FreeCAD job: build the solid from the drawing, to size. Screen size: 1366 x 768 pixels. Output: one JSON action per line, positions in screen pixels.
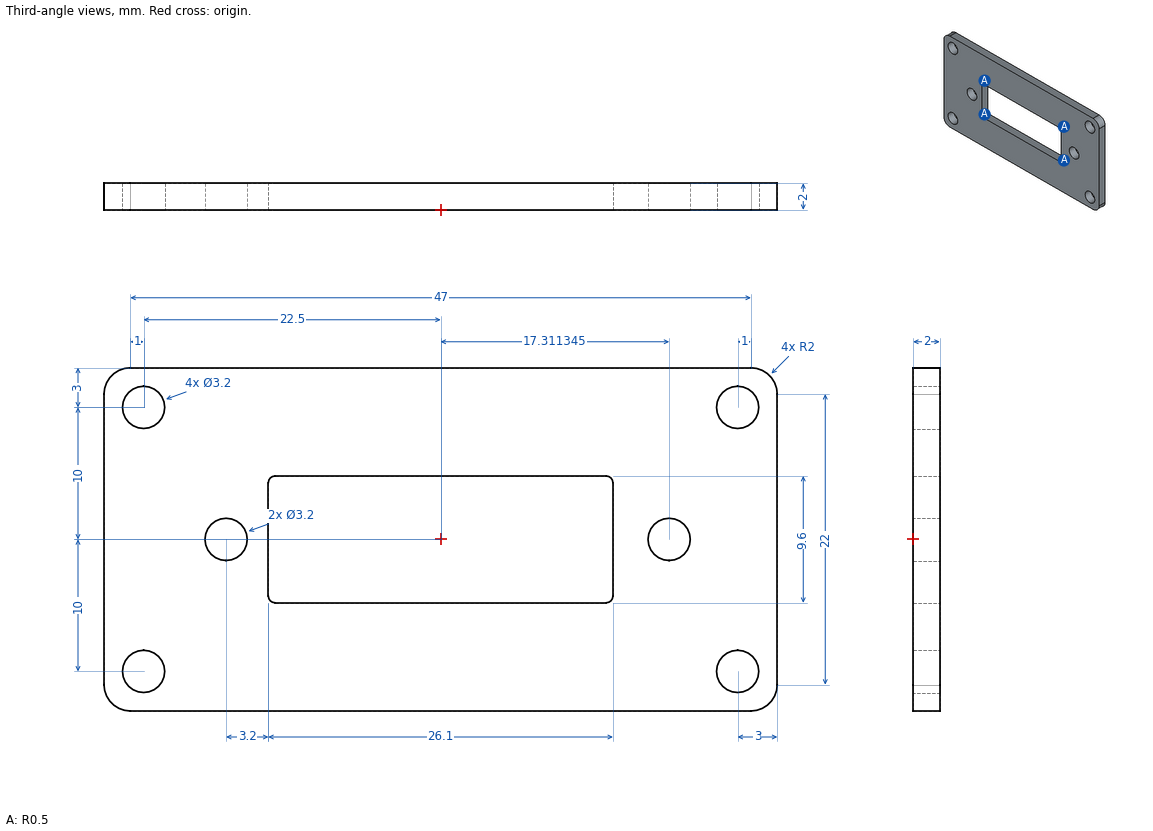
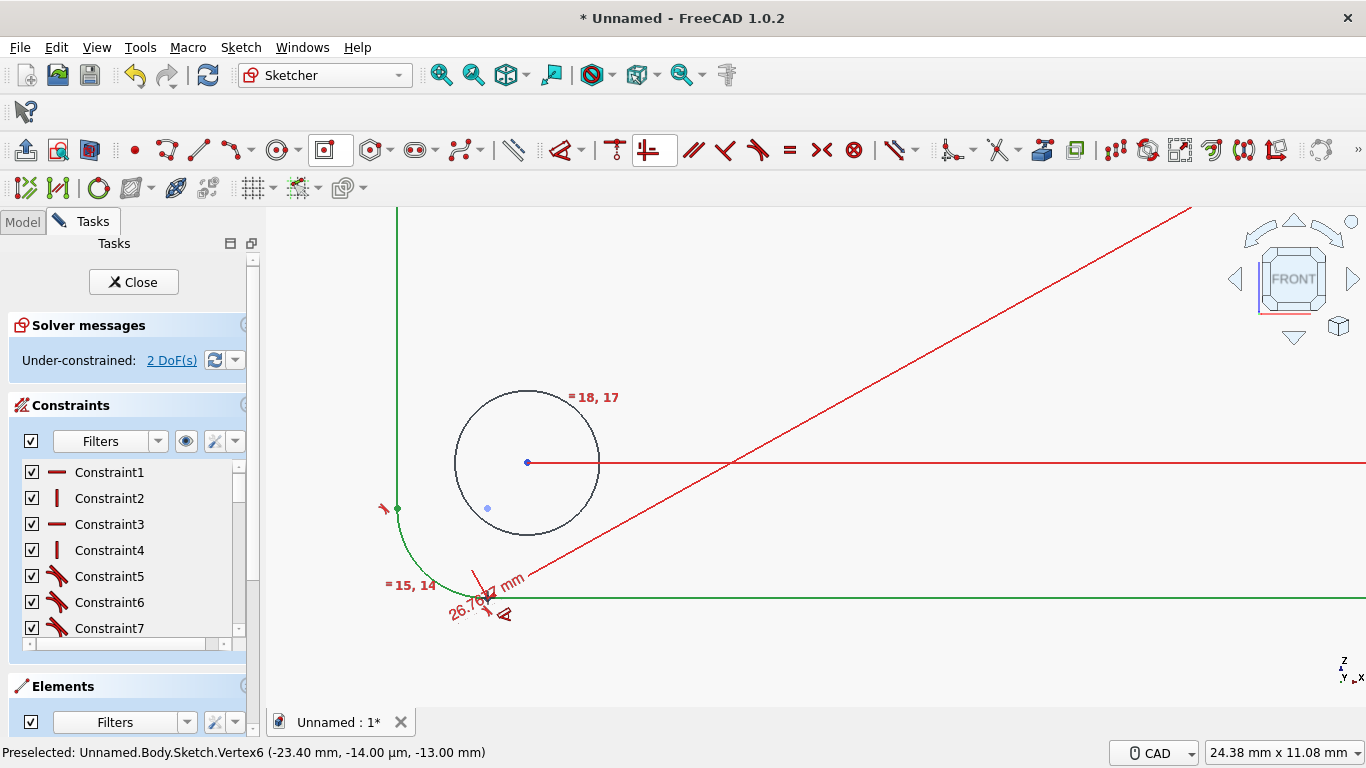
{"action": "left_click", "coordinate": [527, 463]}
{"action": "left_click", "coordinate": [507, 632]}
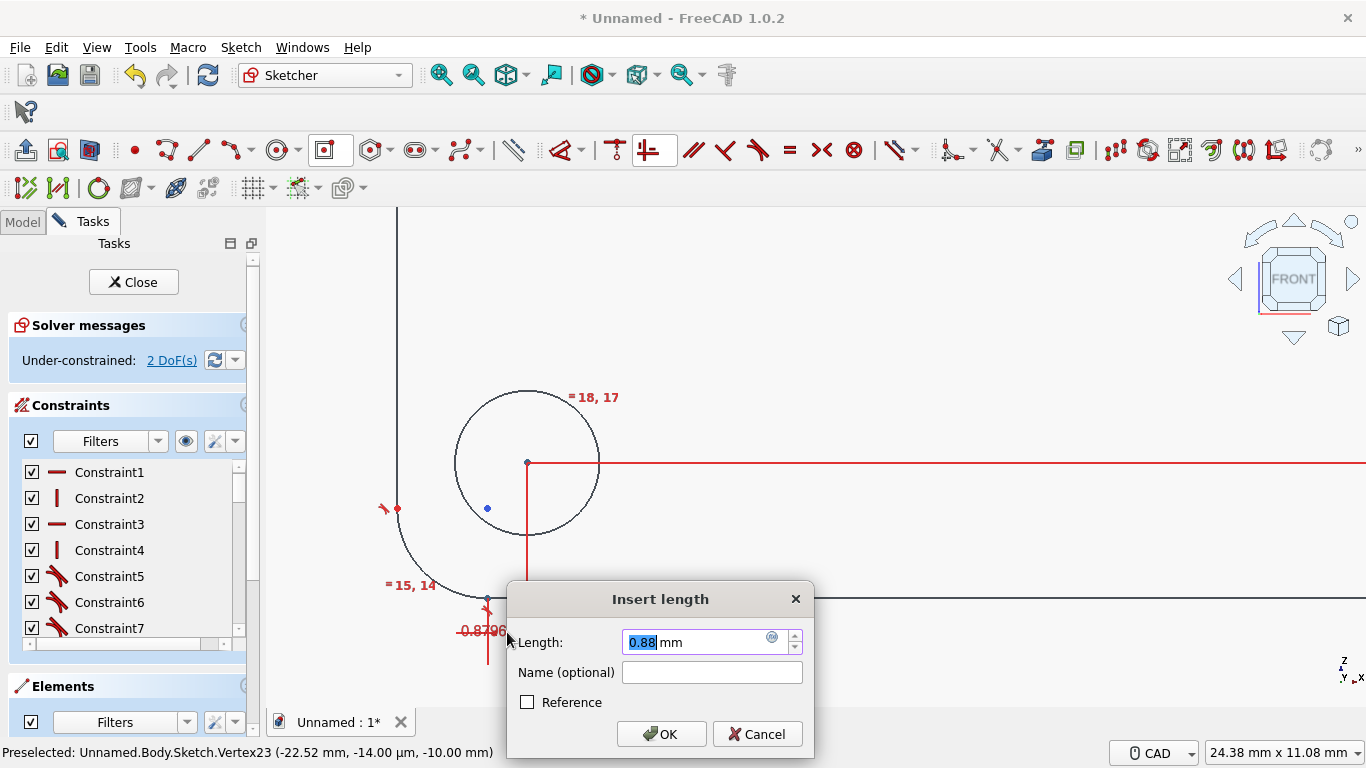
{"action": "type", "text": "1"}
{"action": "key", "text": "Return"}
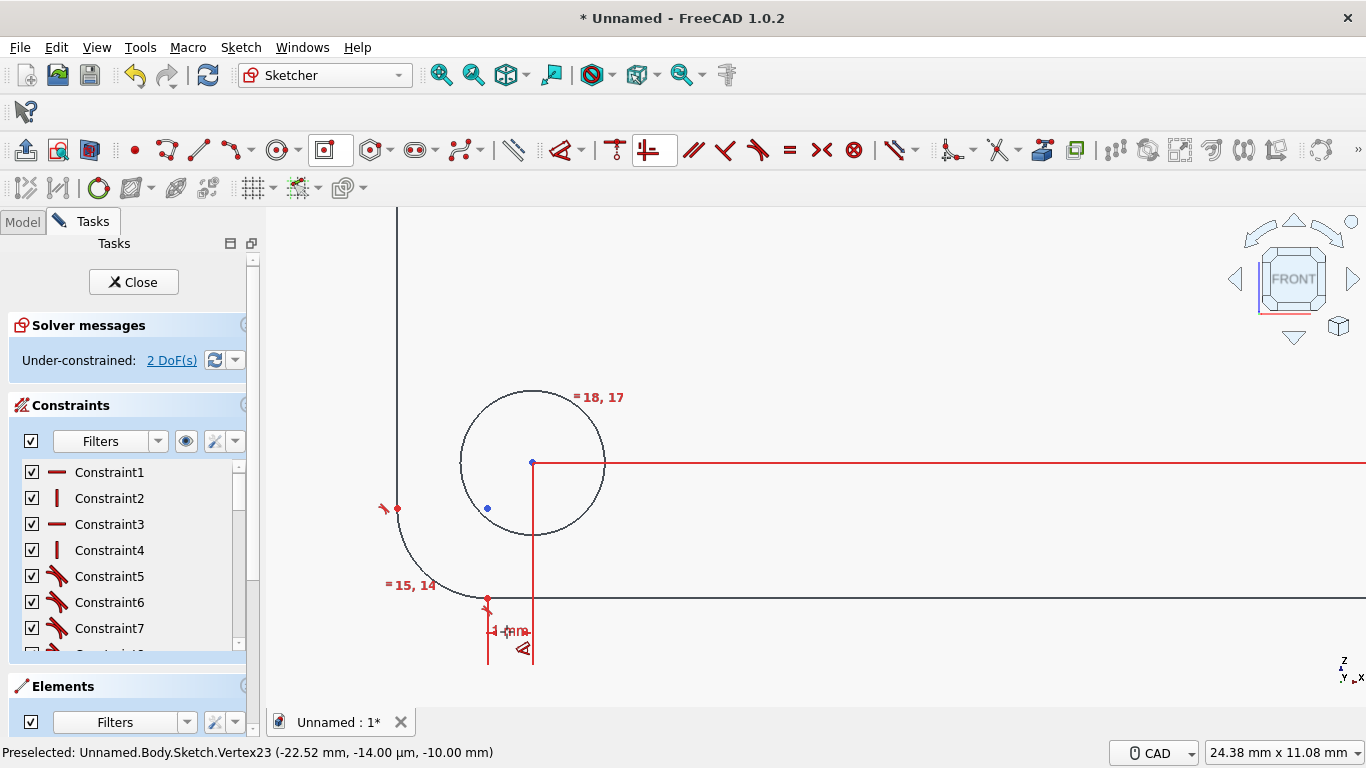
{"action": "scroll", "coordinate": [487, 603], "scroll_direction": "down", "scroll_amount": 7}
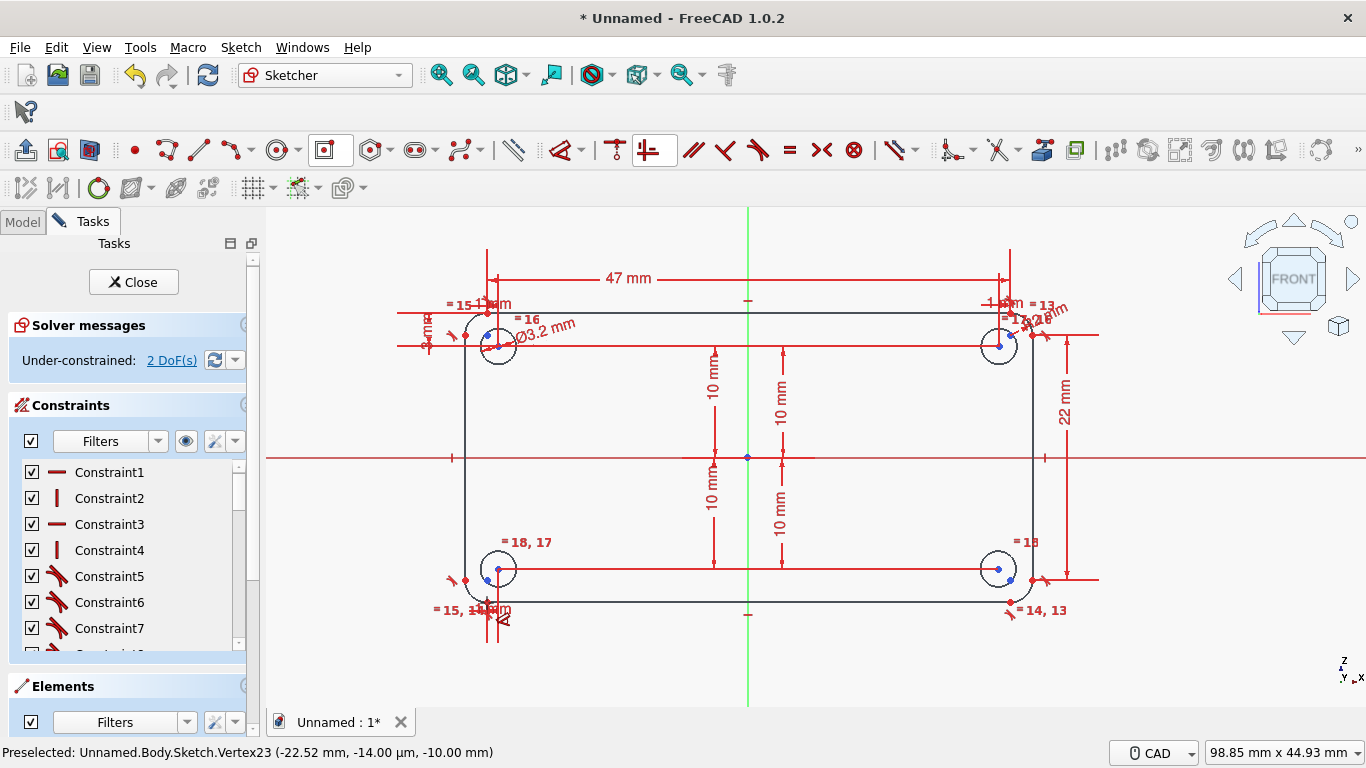
{"action": "left_click", "coordinate": [1033, 580]}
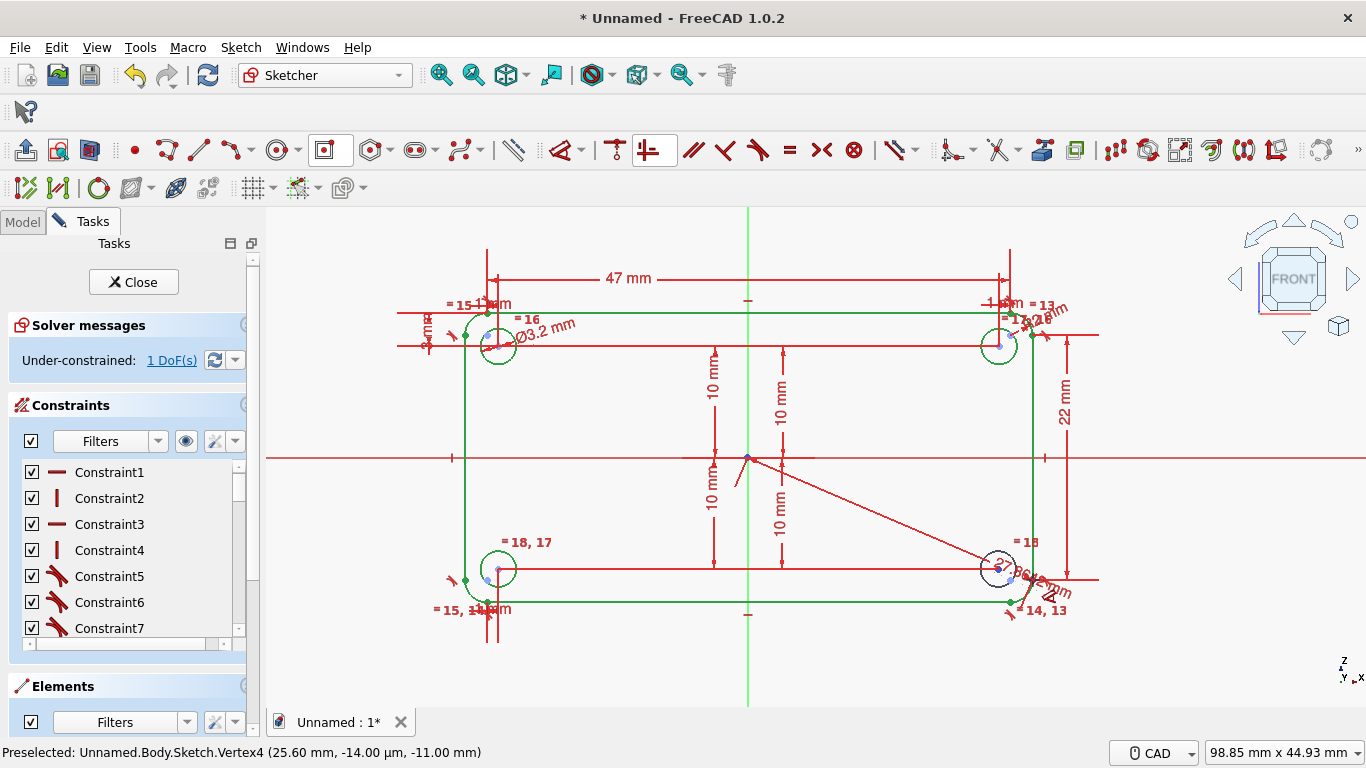
{"action": "left_click", "coordinate": [998, 569]}
{"action": "left_click", "coordinate": [1023, 614]}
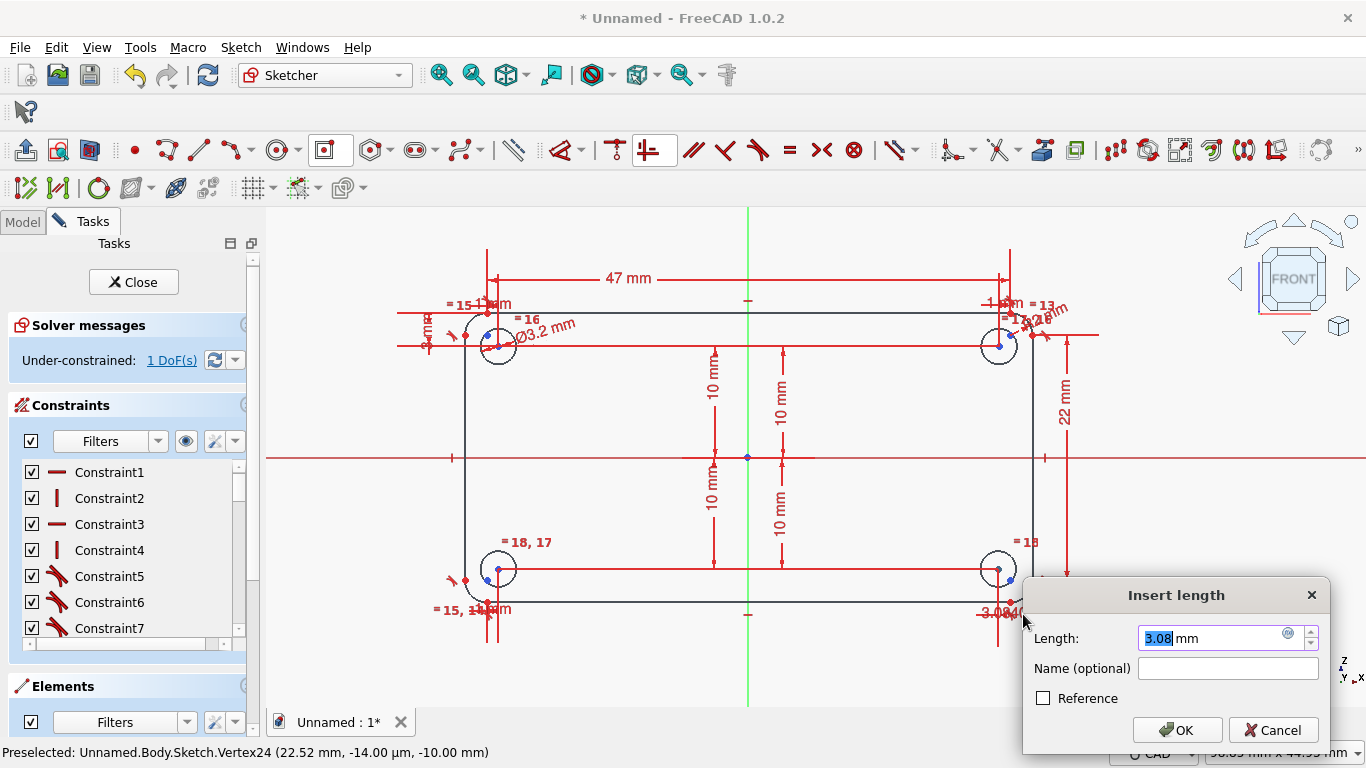
{"action": "type", "text": "3"}
{"action": "key", "text": "Return"}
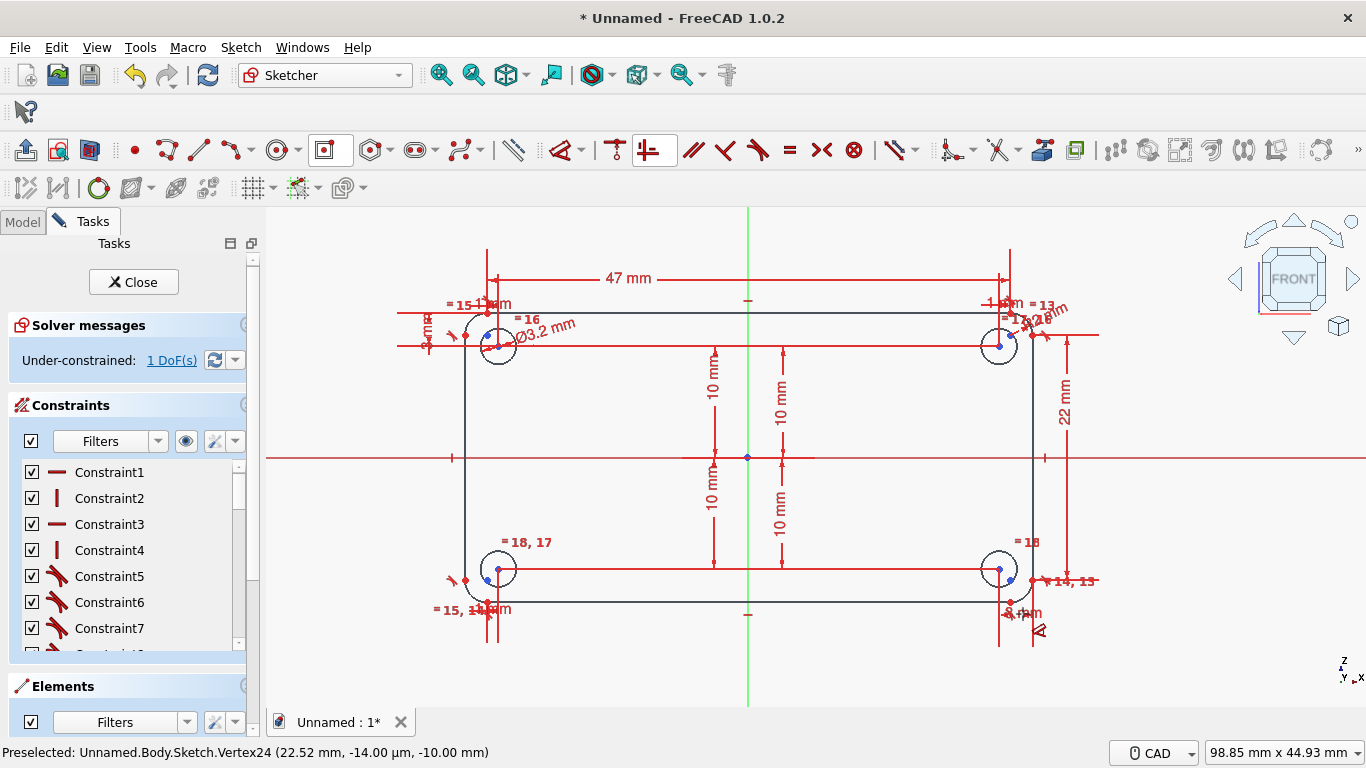
{"action": "left_click", "coordinate": [498, 346]}
{"action": "left_click", "coordinate": [623, 492]}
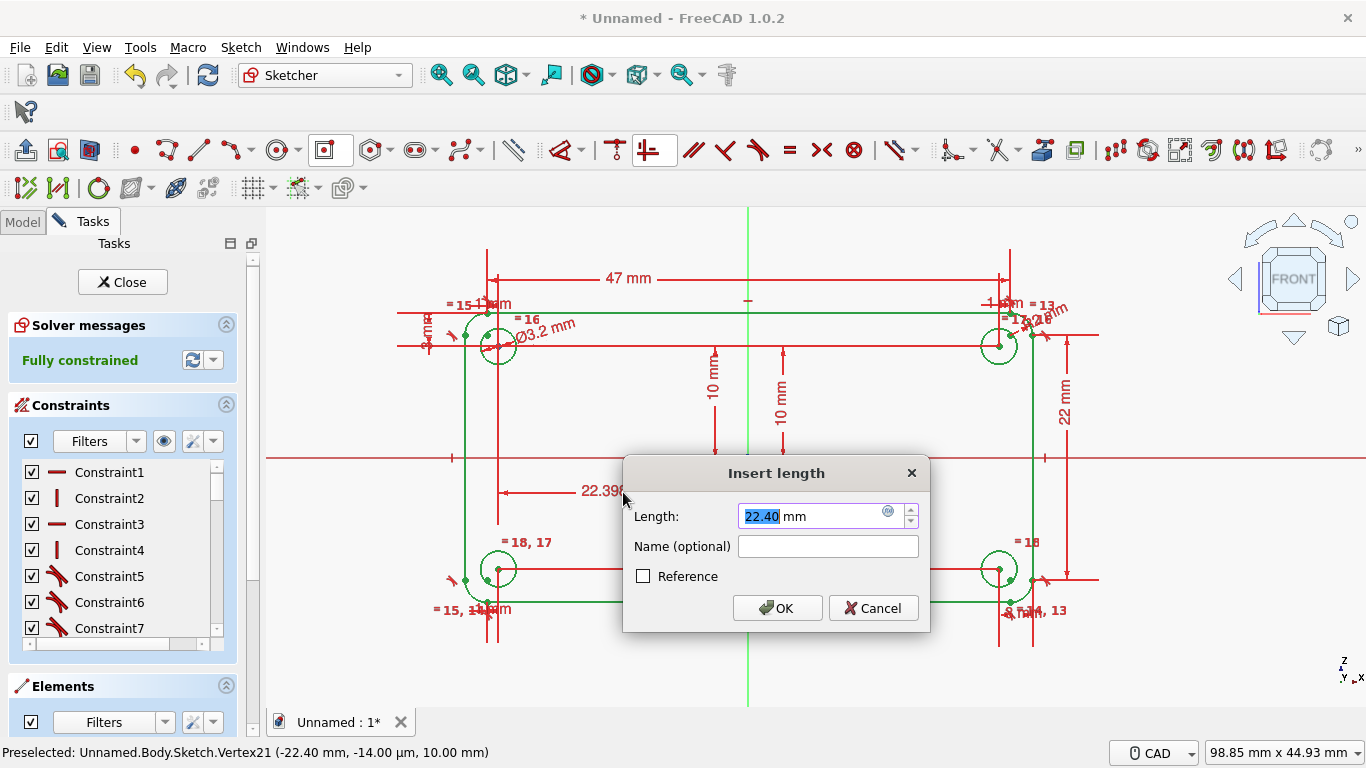
{"action": "type", "text": "22.5"}
{"action": "key", "text": "Return"}
{"action": "key", "text": "Escape"}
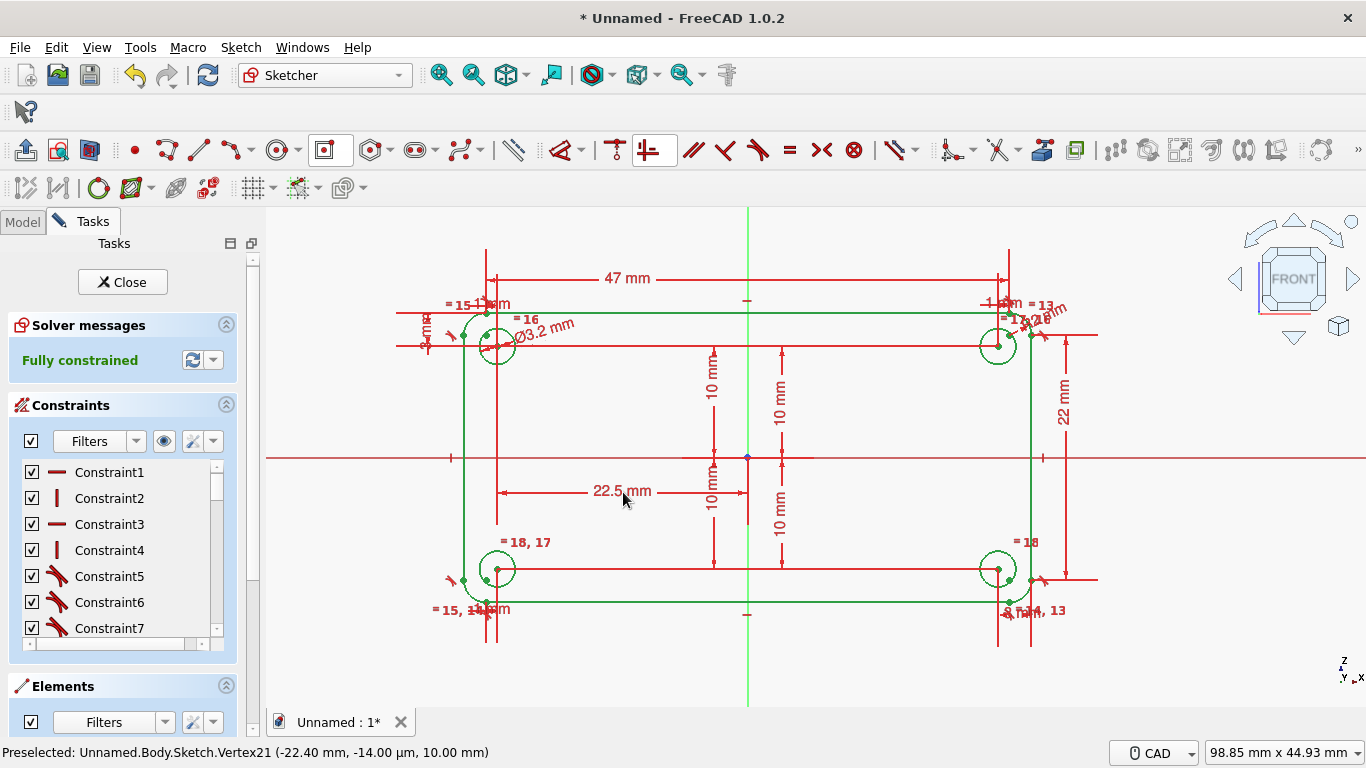
{"action": "left_click", "coordinate": [123, 282]}